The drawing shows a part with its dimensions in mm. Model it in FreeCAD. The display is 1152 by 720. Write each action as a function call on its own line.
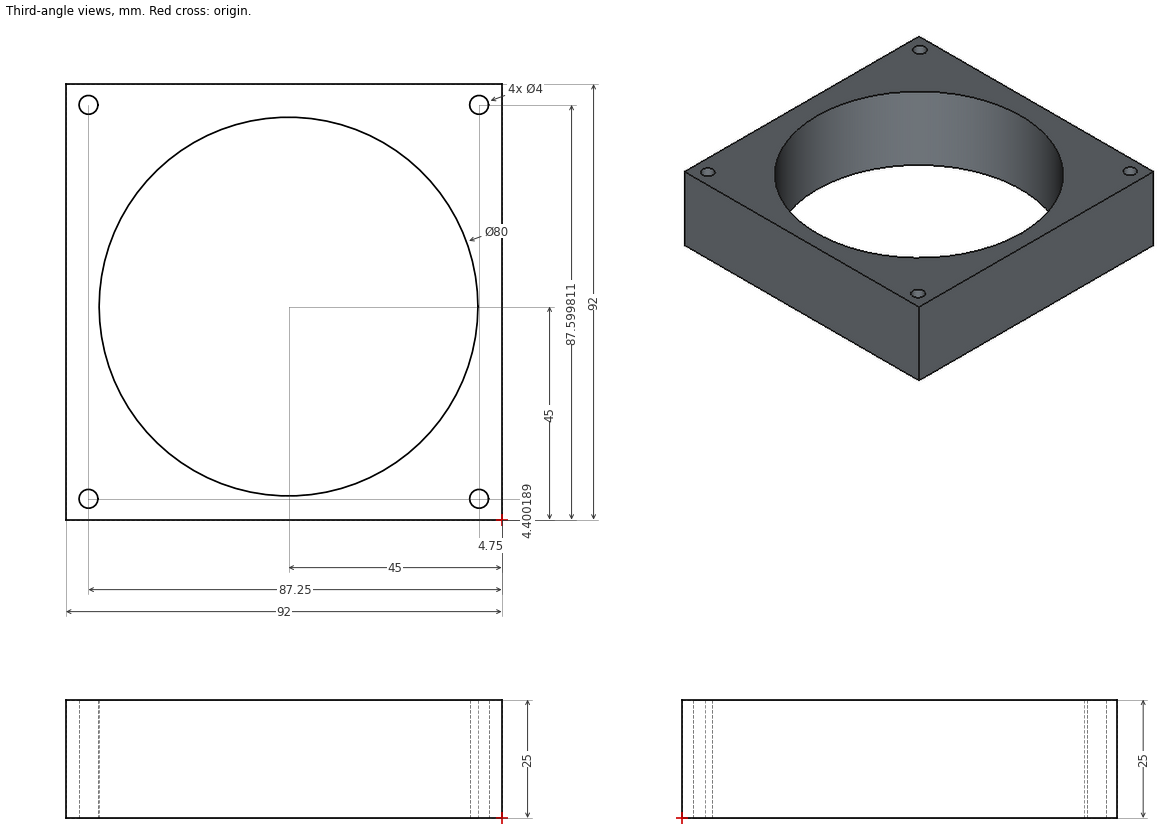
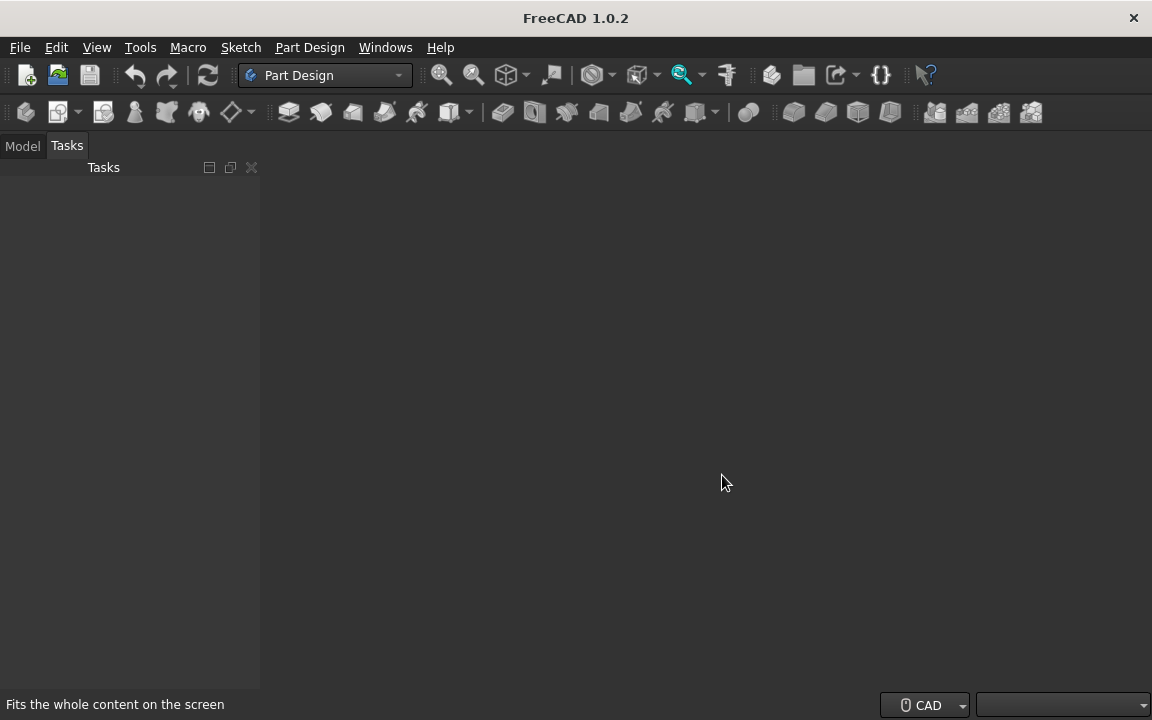
key(ctrl+n)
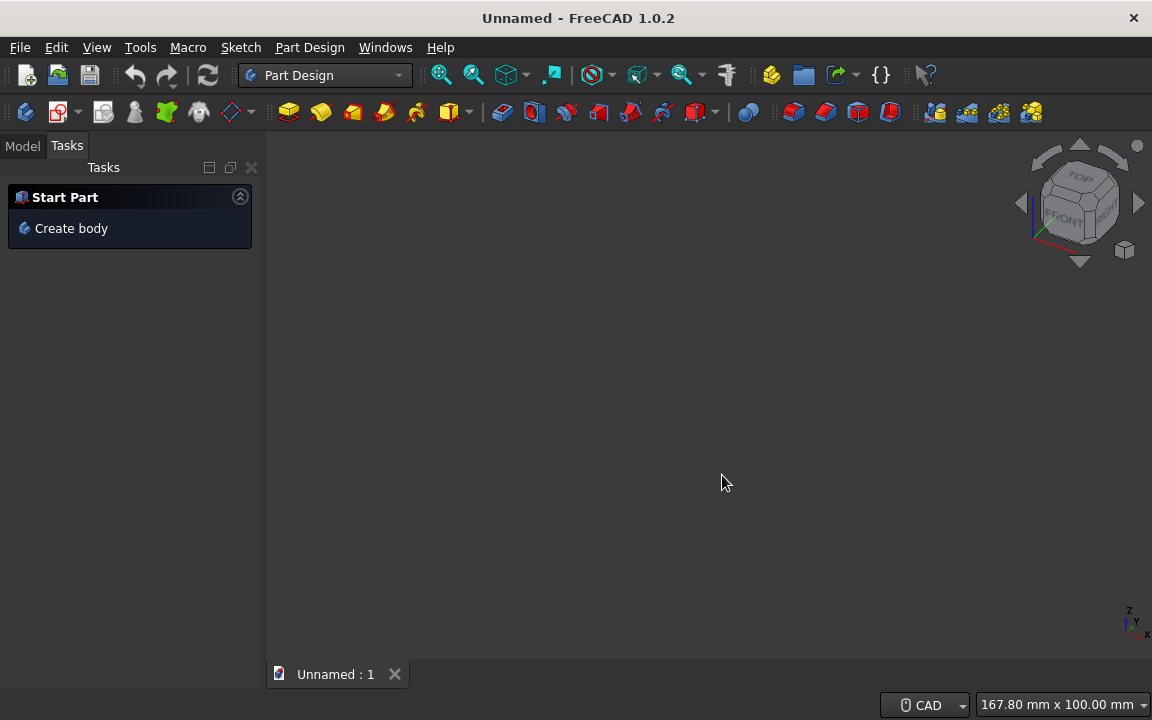
click(58, 112)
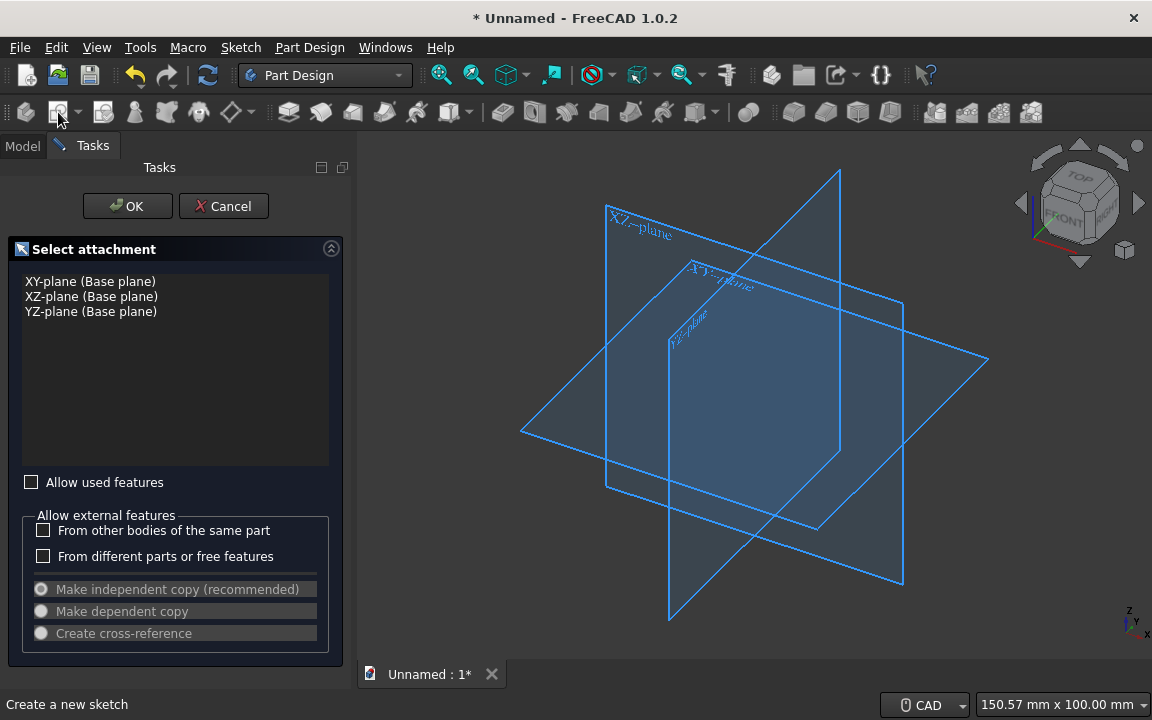
click(82, 282)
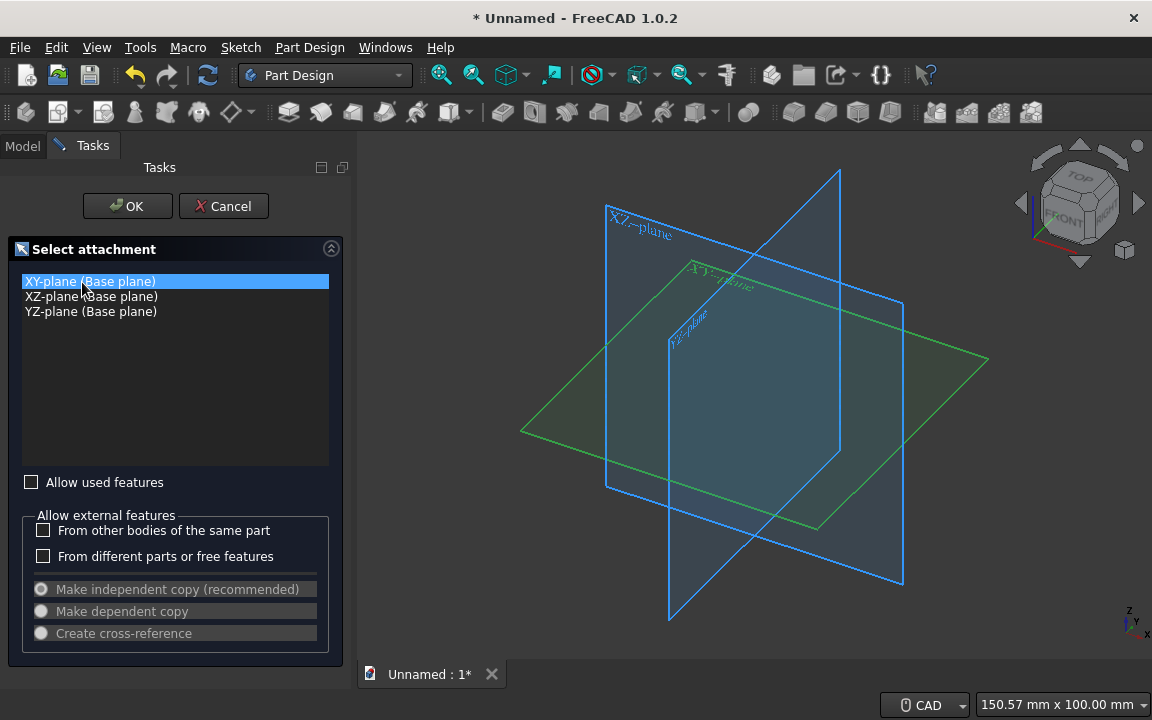
click(128, 206)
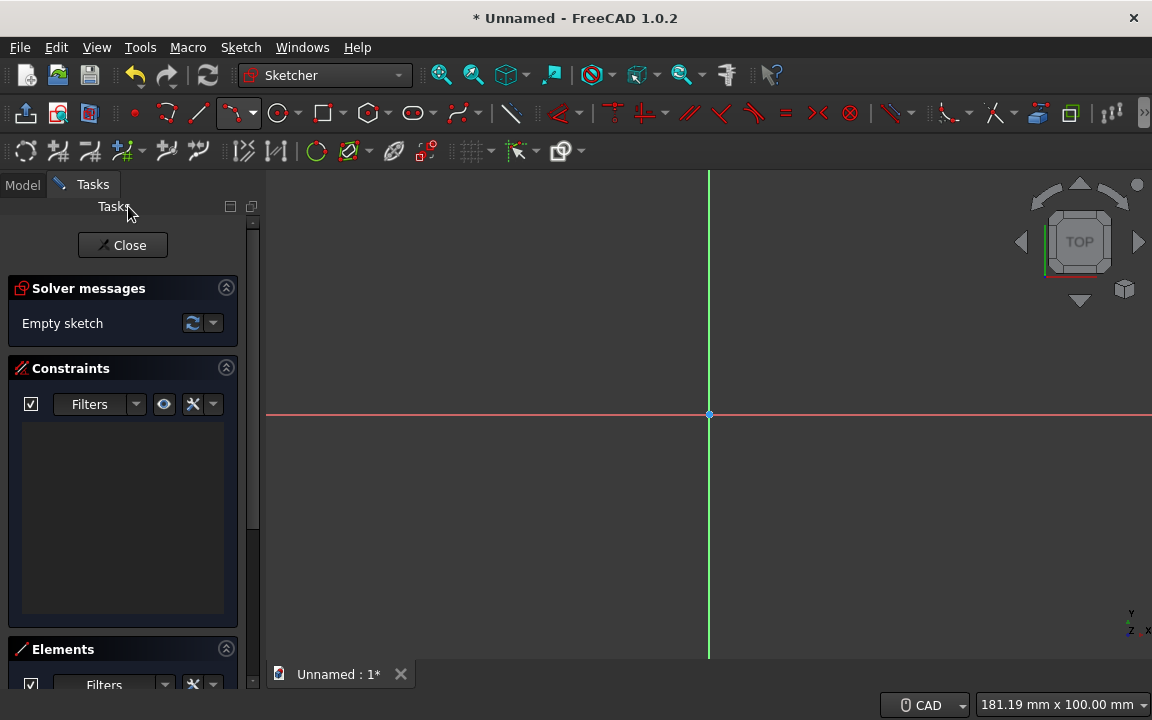
scroll(831, 631, down, 3)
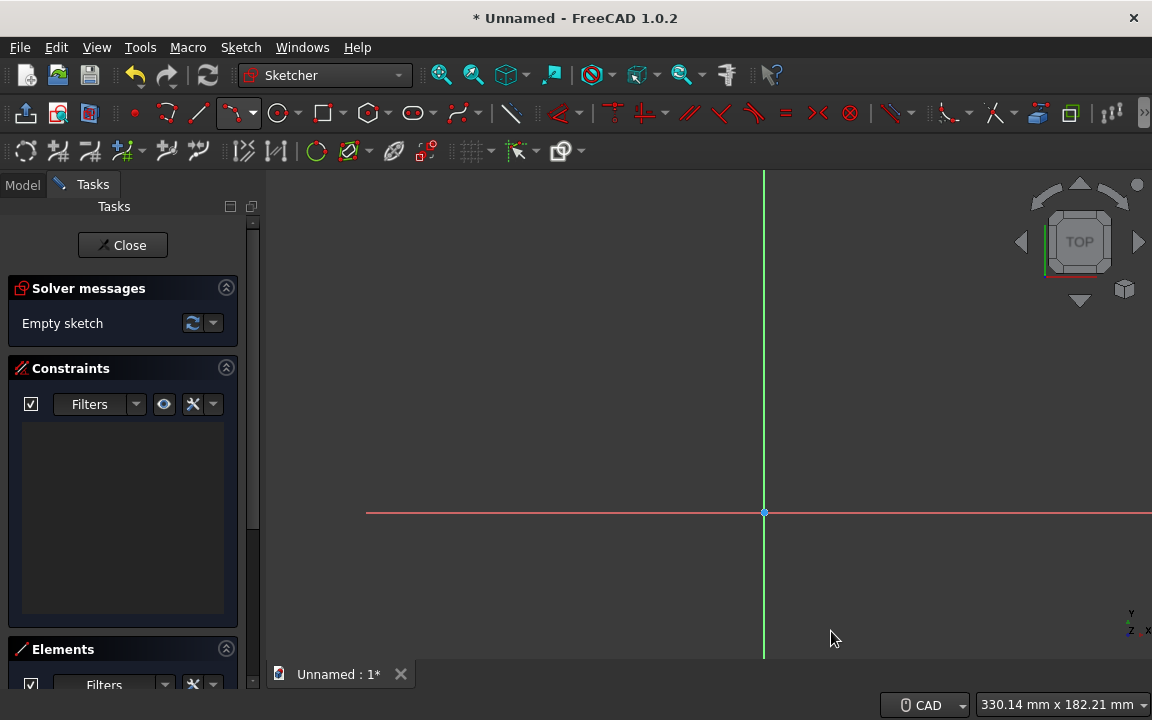
key(g)
key(r)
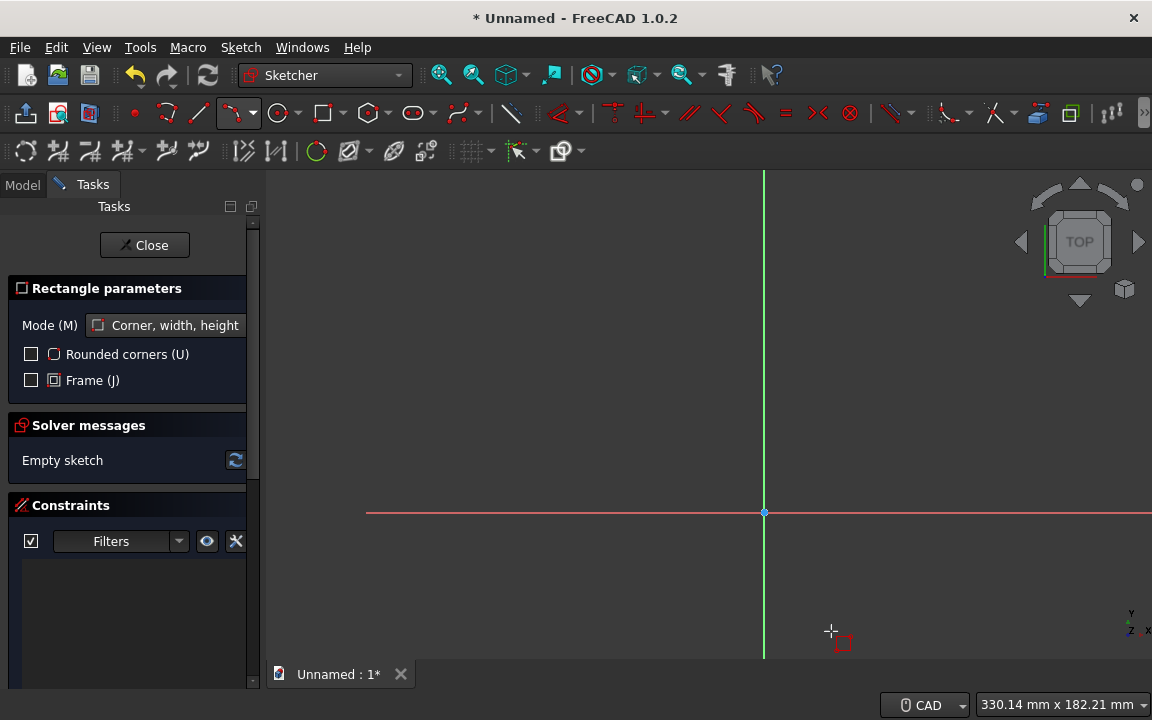
click(764, 513)
move(517, 266)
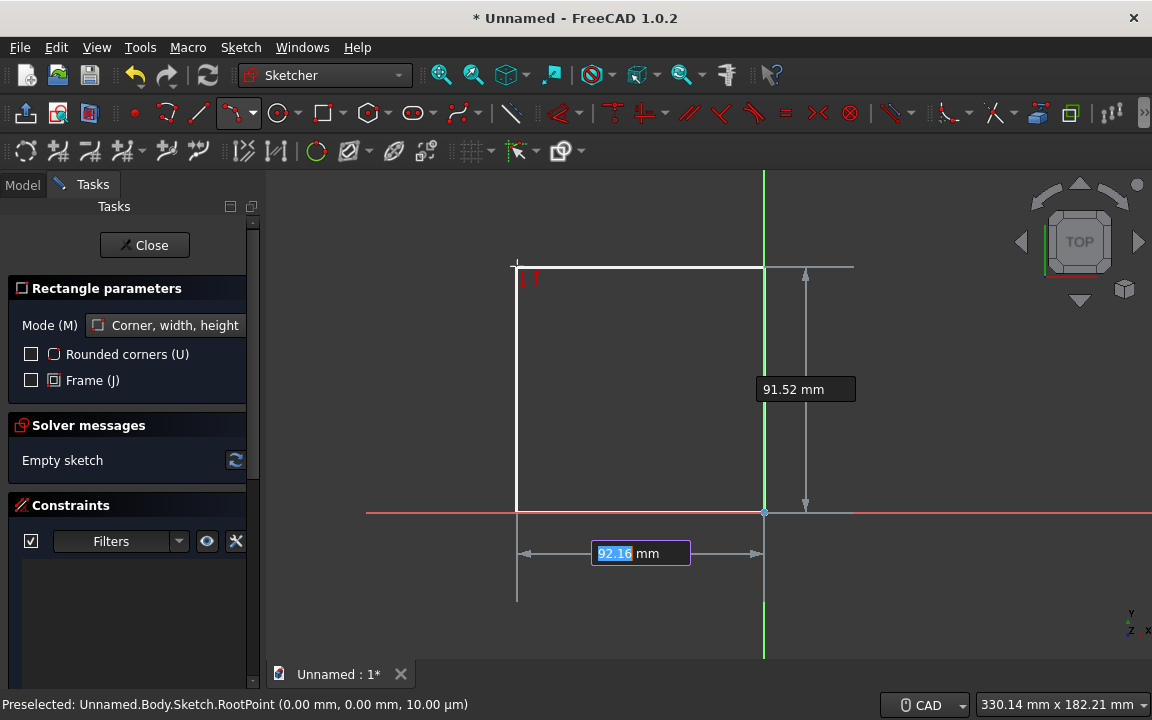
text(92)
key(Tab)
text(92)
key(Return)
key(Escape)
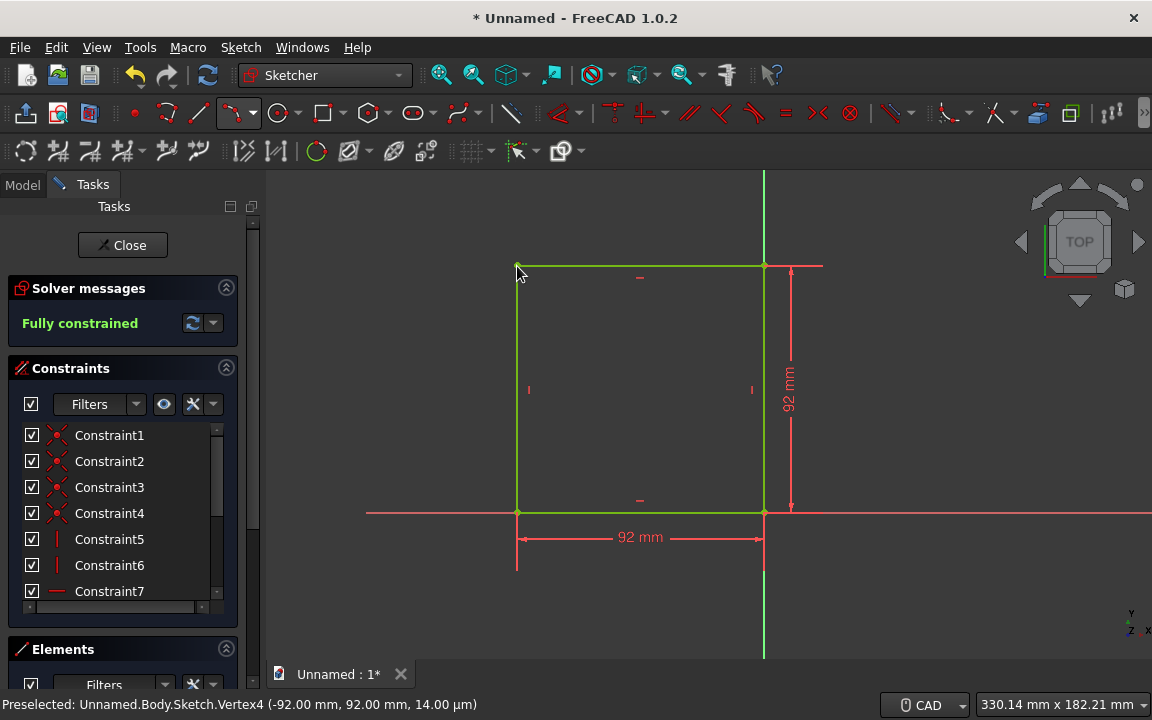
click(123, 245)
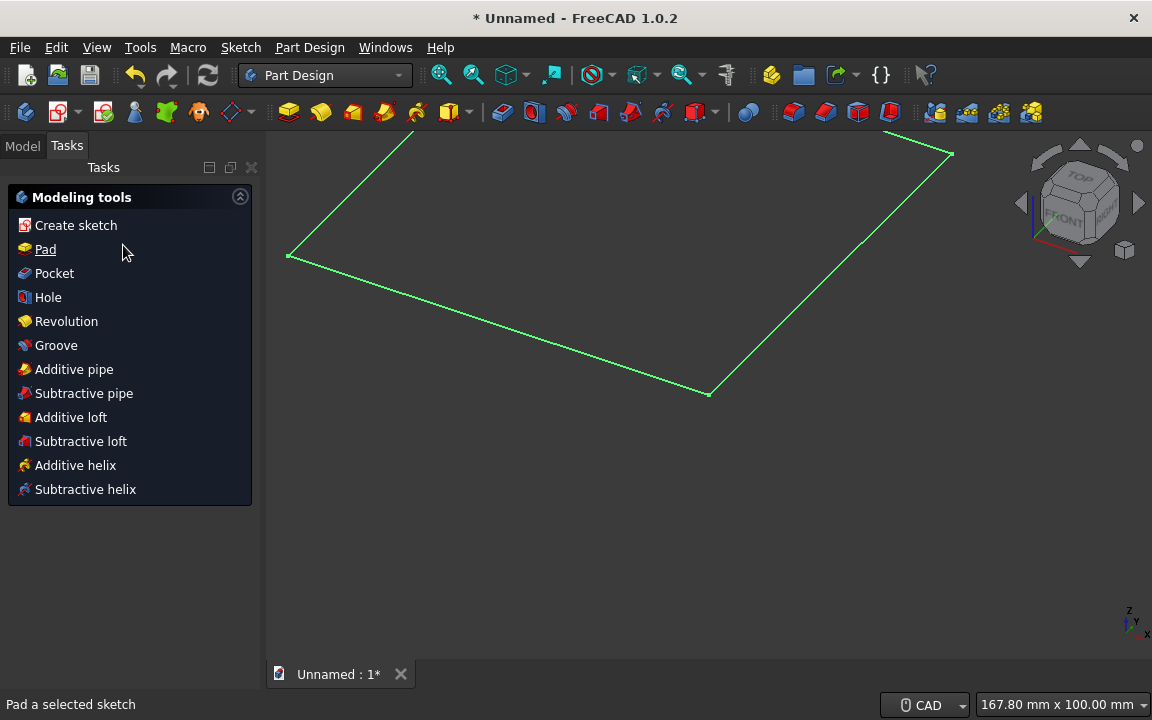
click(290, 112)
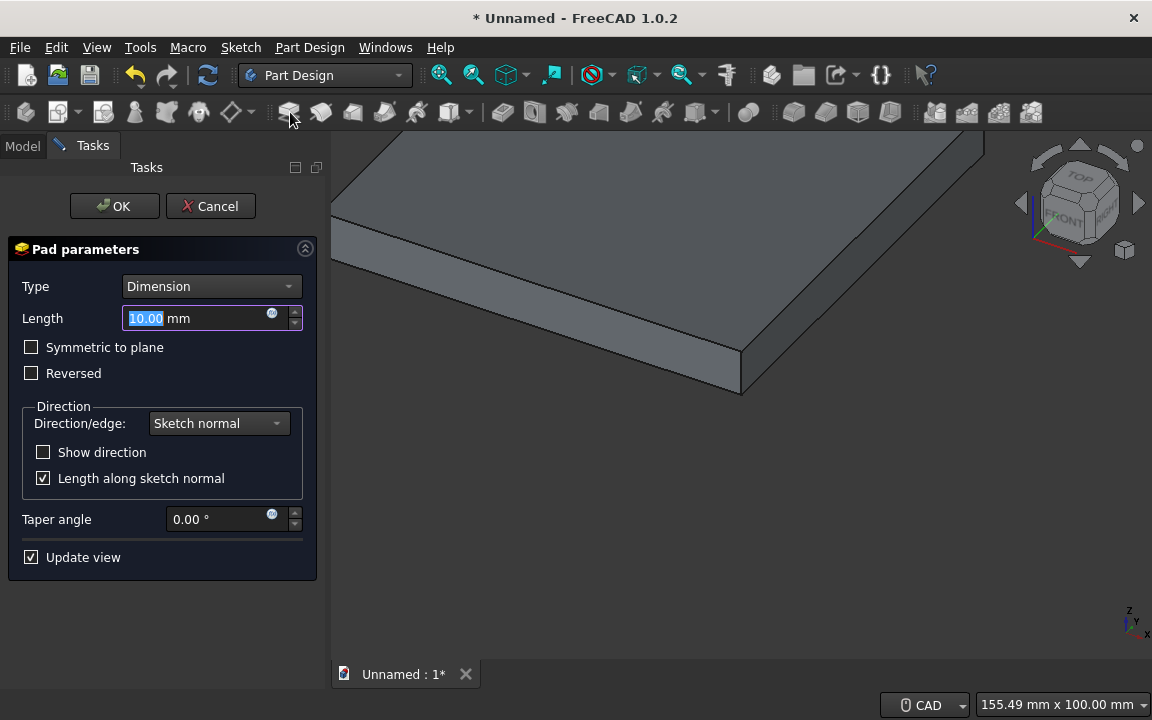
text(25)
key(Tab)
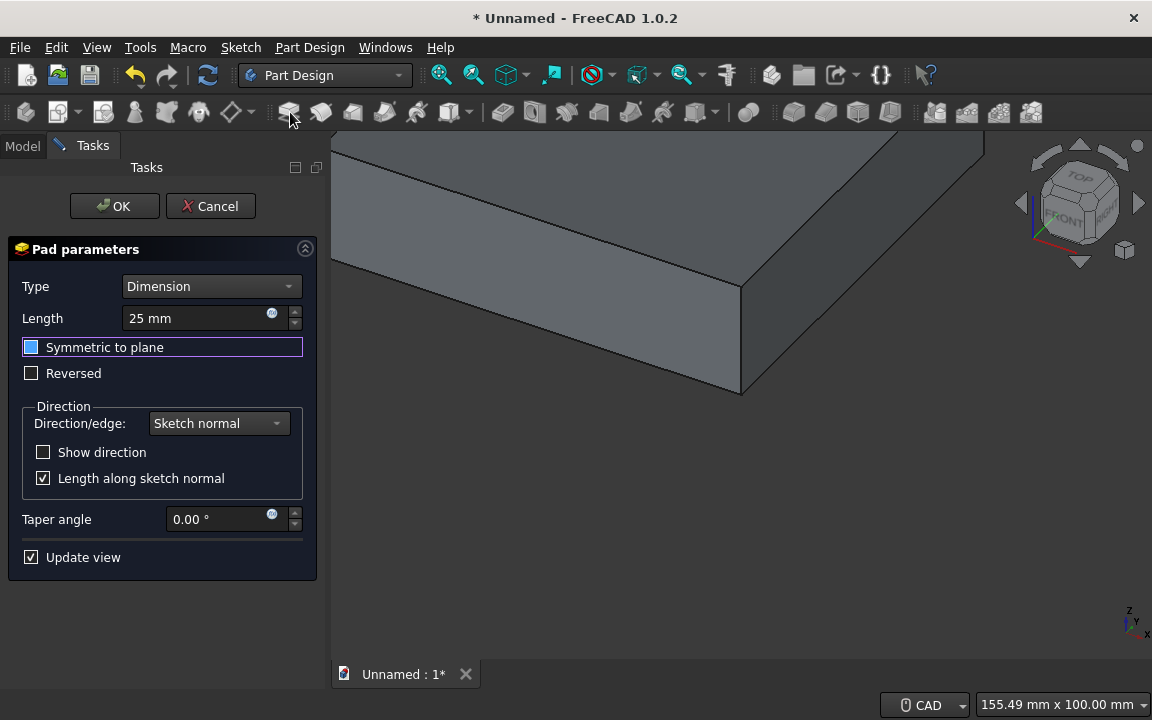
click(115, 206)